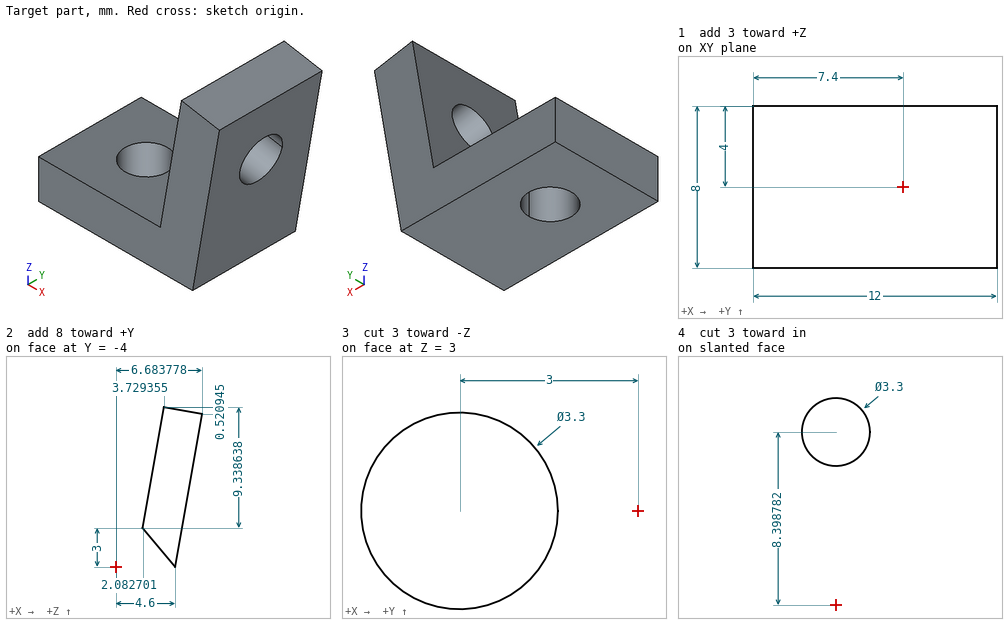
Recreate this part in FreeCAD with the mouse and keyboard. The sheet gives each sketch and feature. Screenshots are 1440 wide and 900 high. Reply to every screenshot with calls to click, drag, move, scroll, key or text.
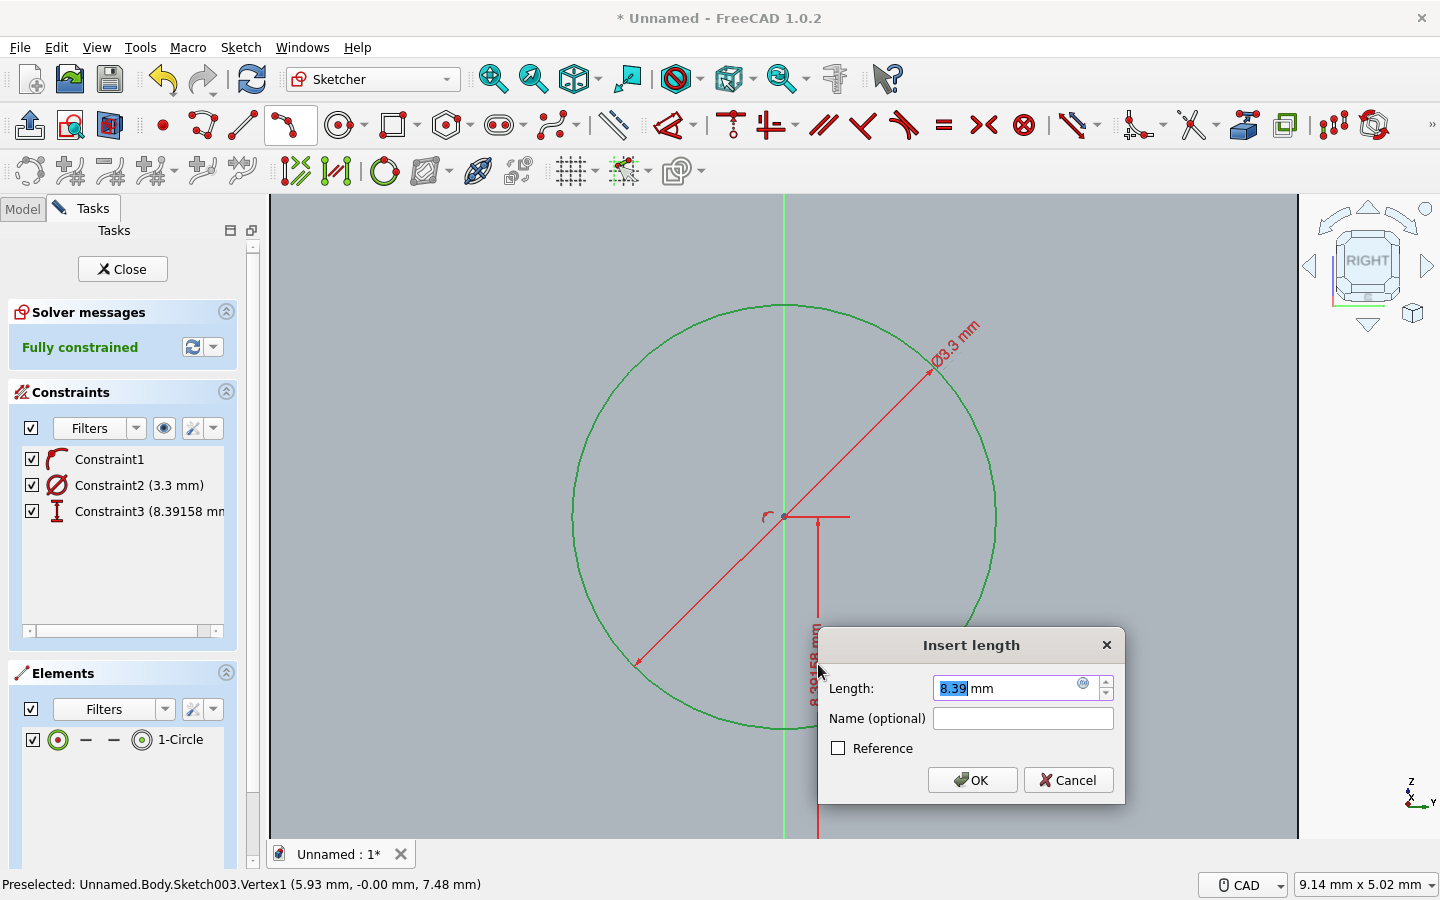
text(8.398782)
key(Return)
key(Escape)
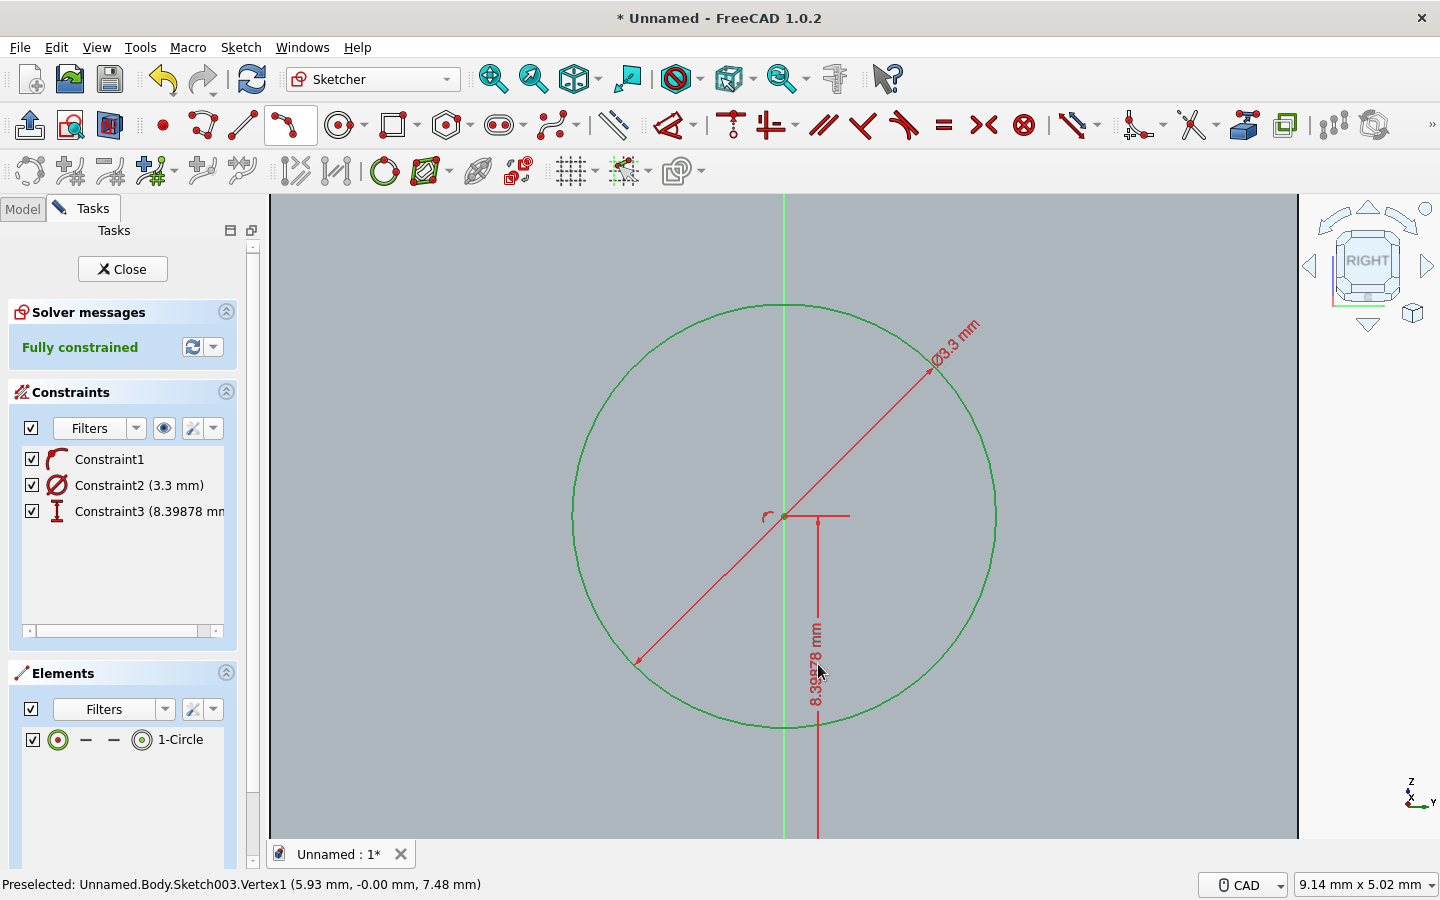
click(123, 269)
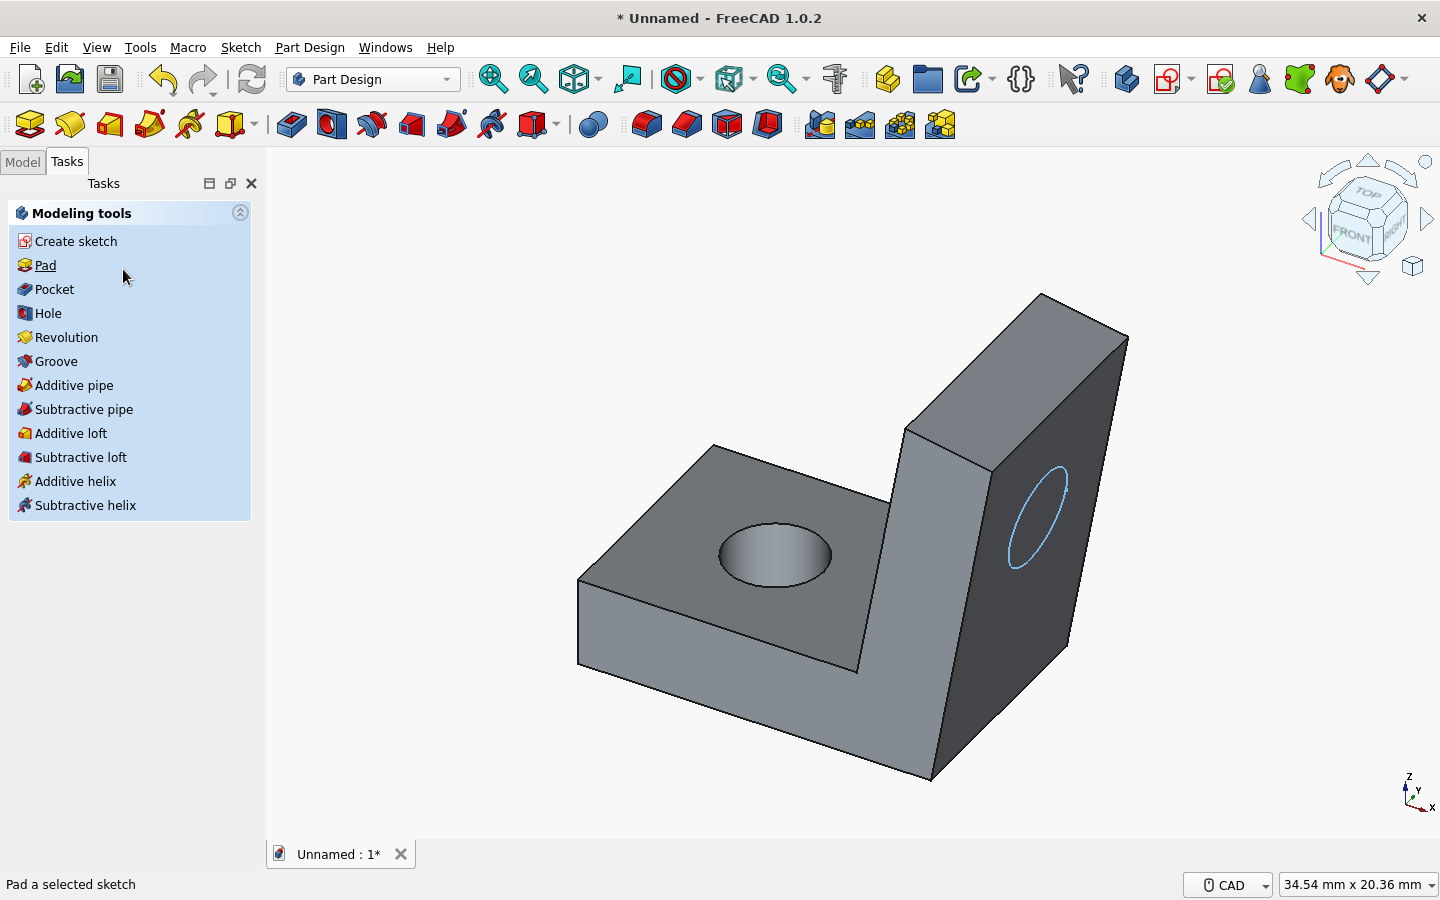
click(292, 124)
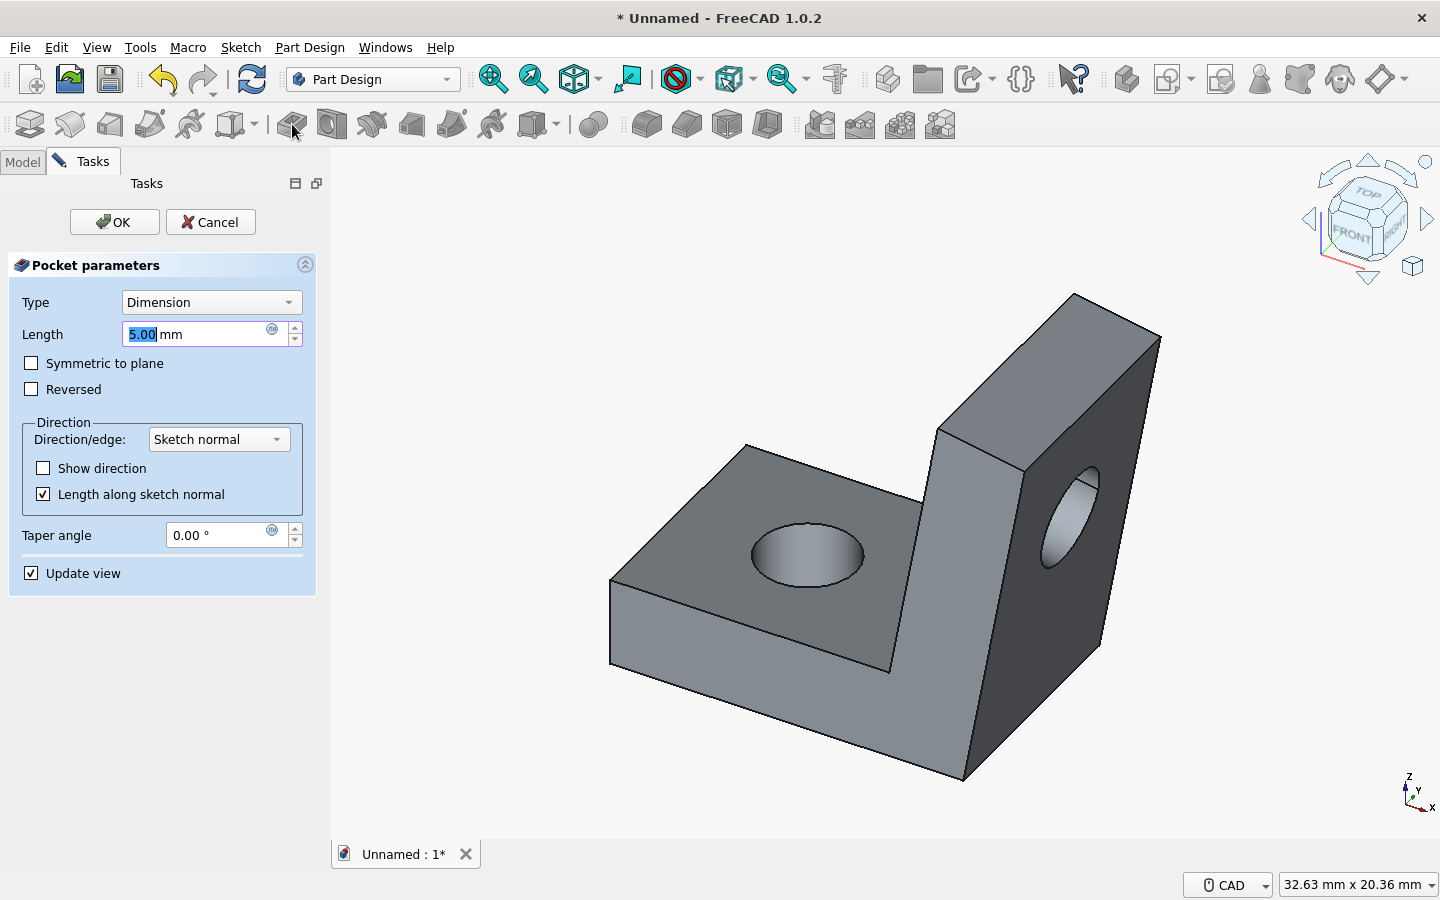
text(3)
key(Tab)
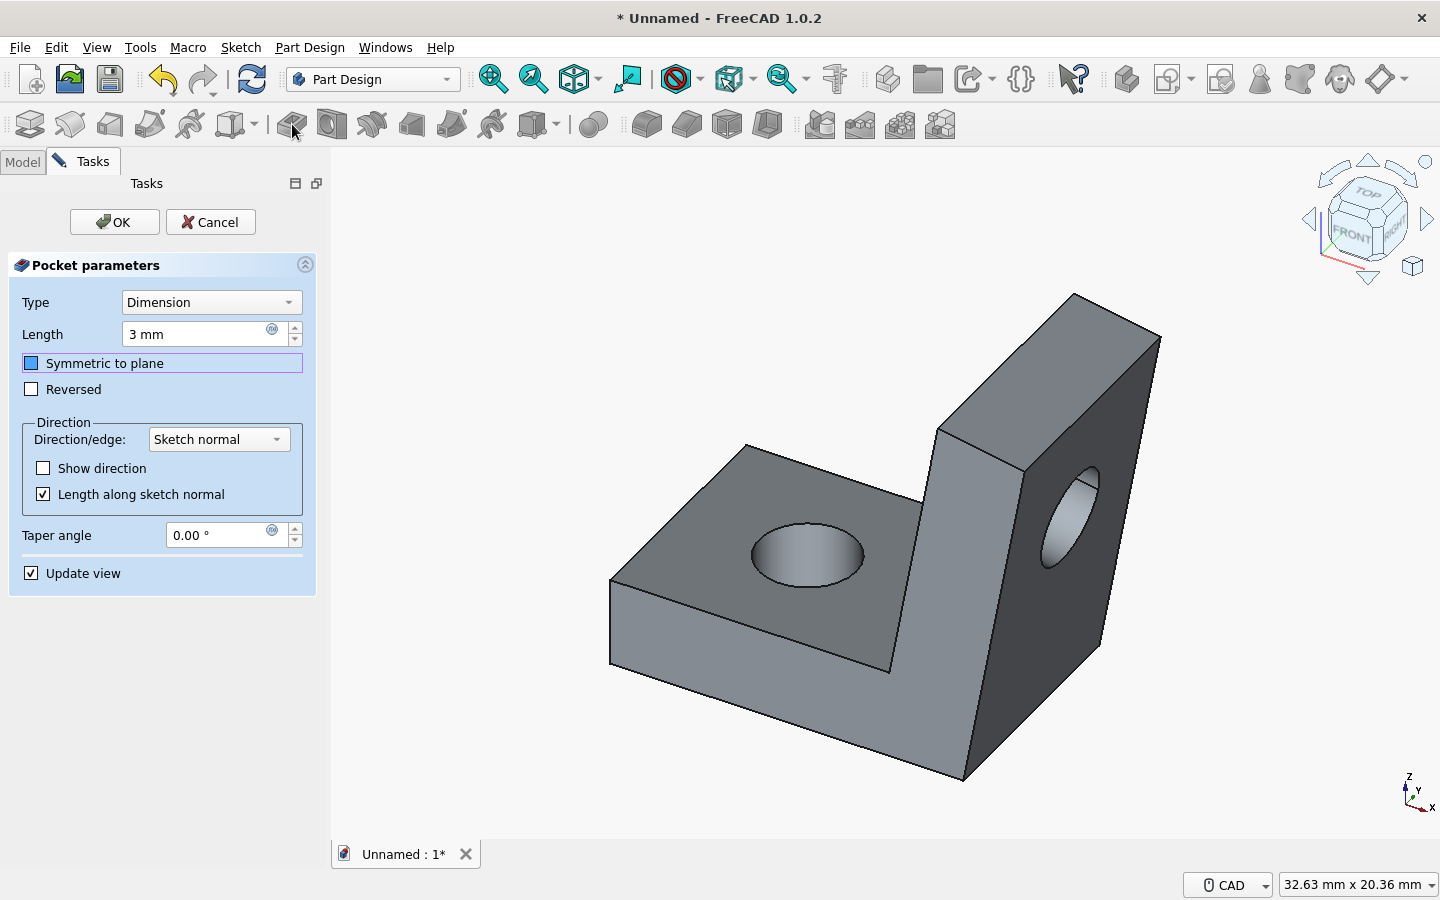
click(115, 222)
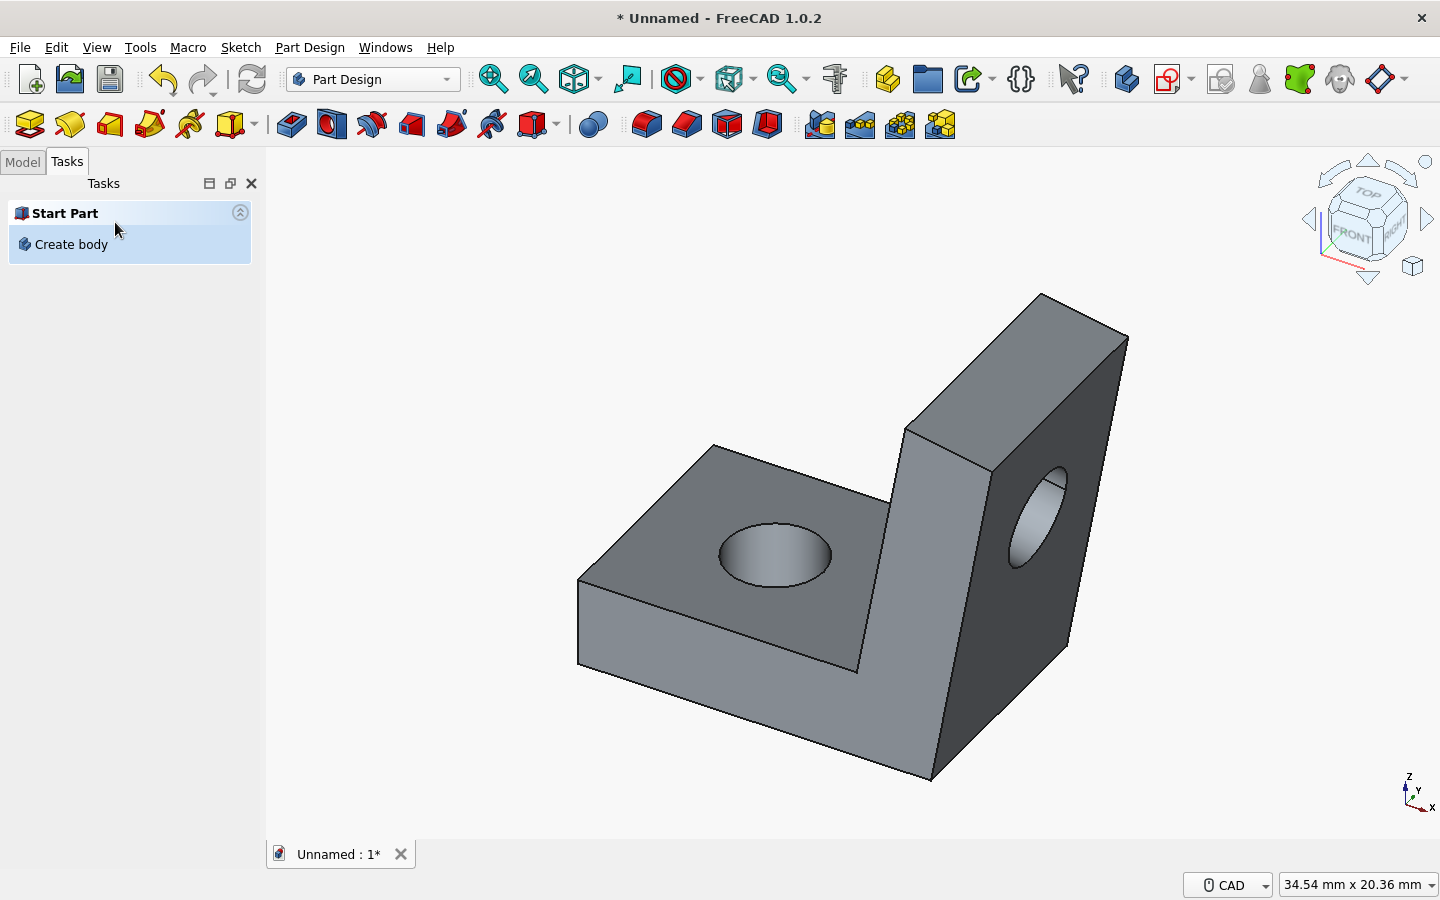
key(0)